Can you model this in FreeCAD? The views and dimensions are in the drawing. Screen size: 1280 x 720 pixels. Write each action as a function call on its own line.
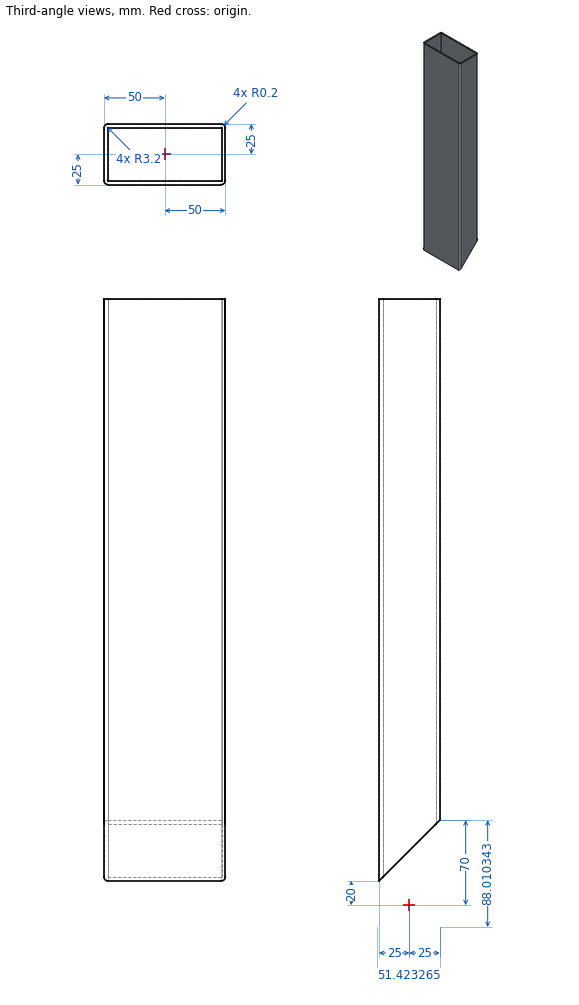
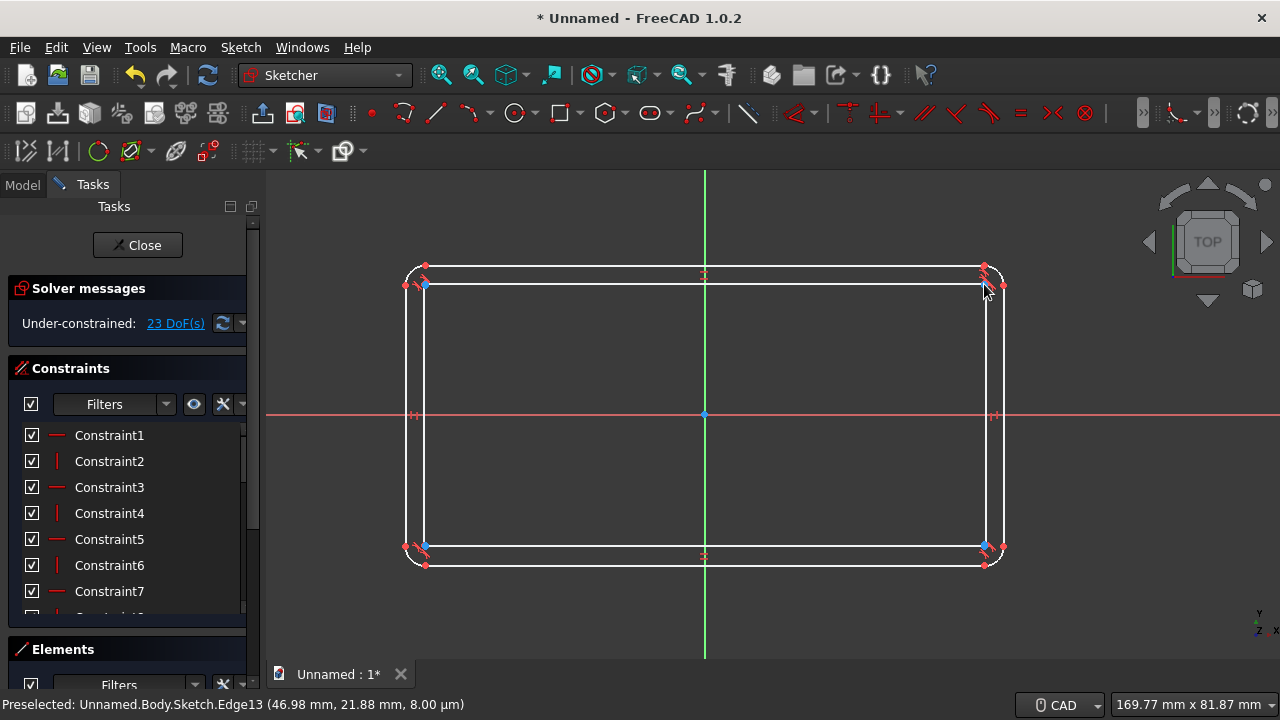
click(593, 284)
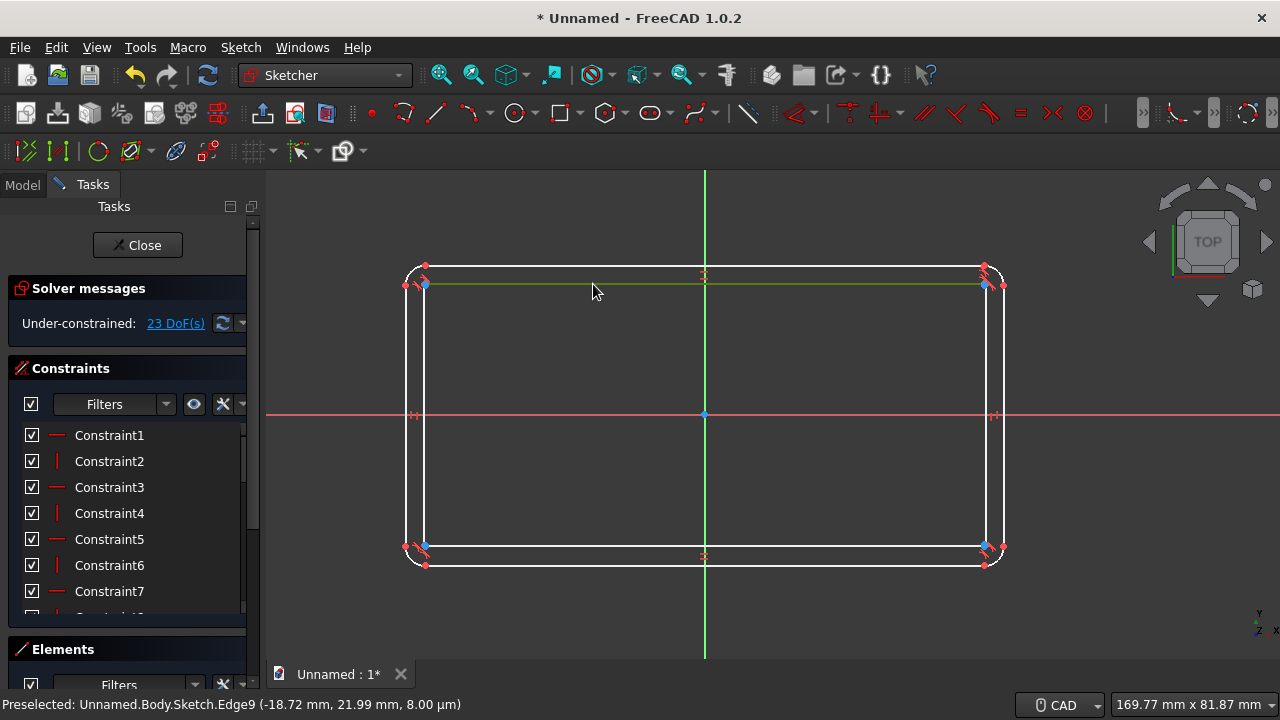
scroll(424, 284, up, 13)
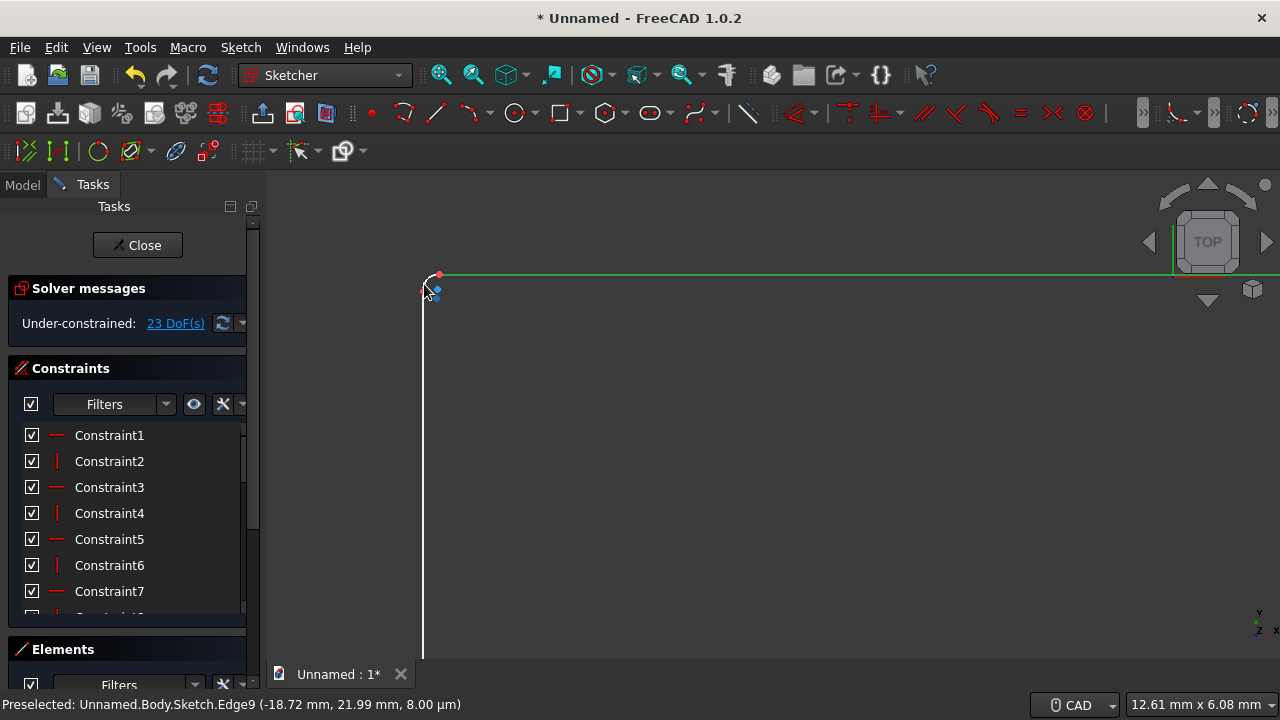
click(427, 279)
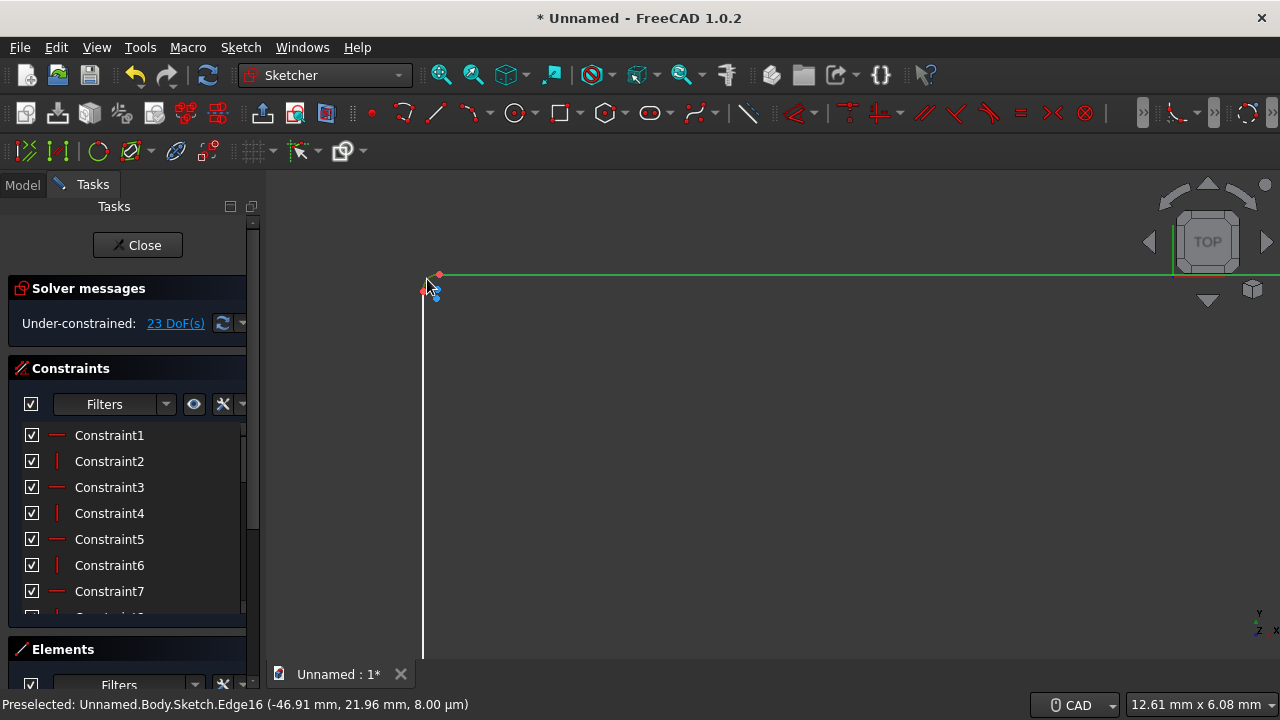
click(990, 114)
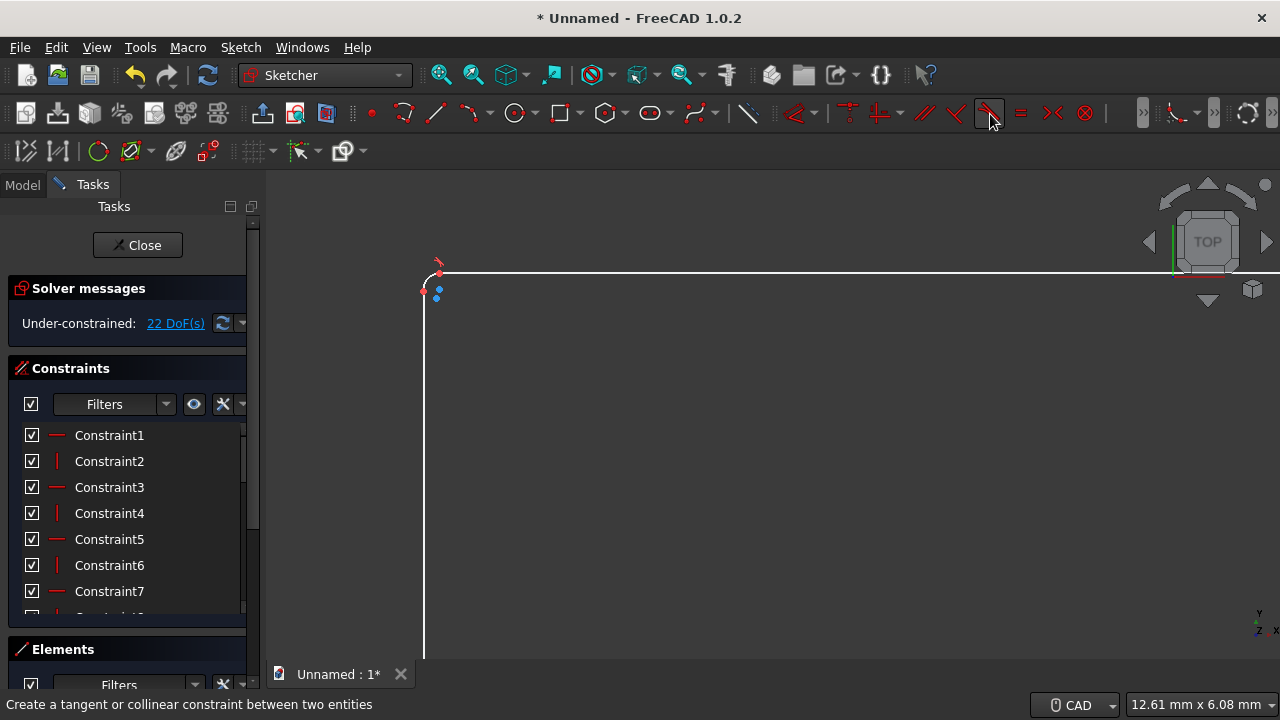
scroll(424, 284, down, 13)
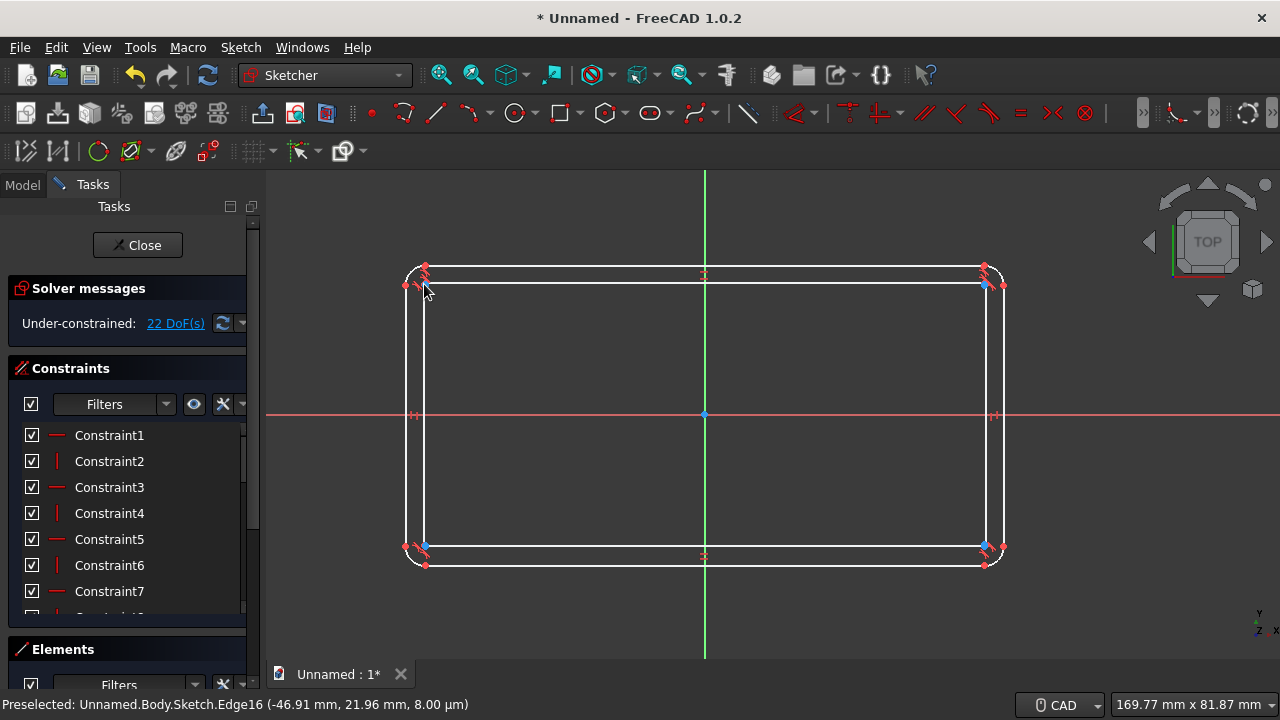
click(986, 363)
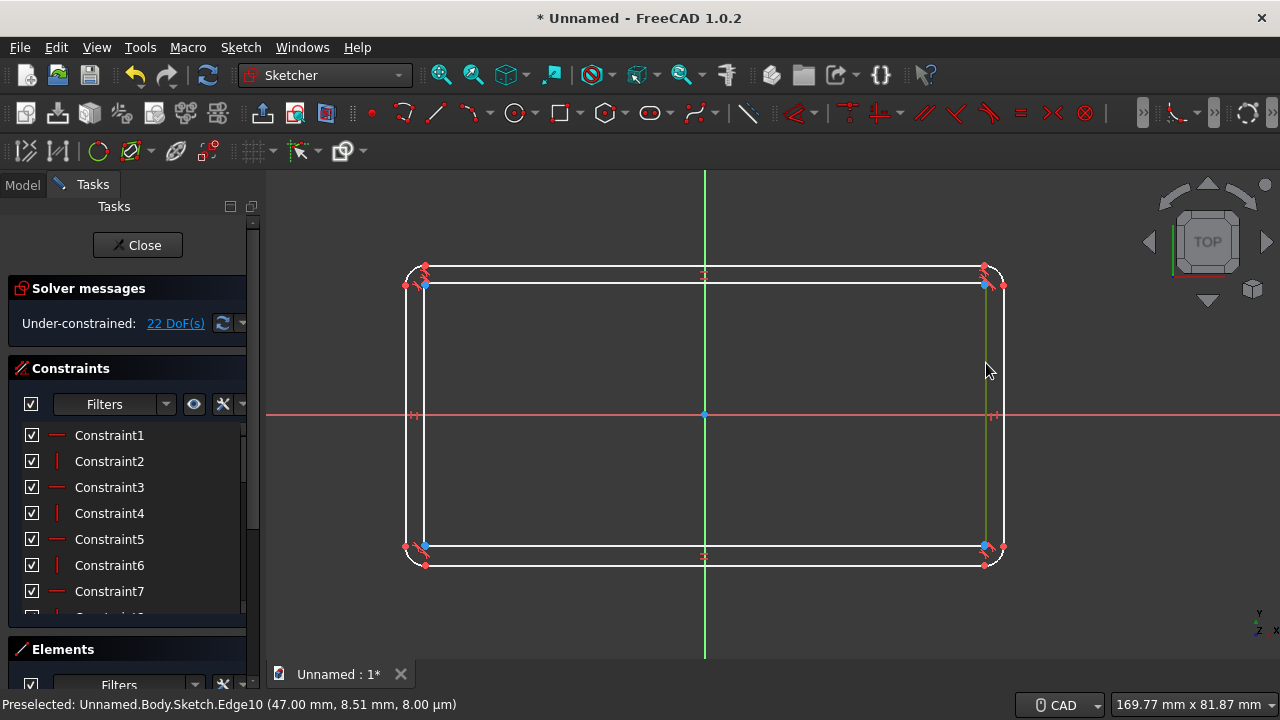
scroll(985, 284, up, 13)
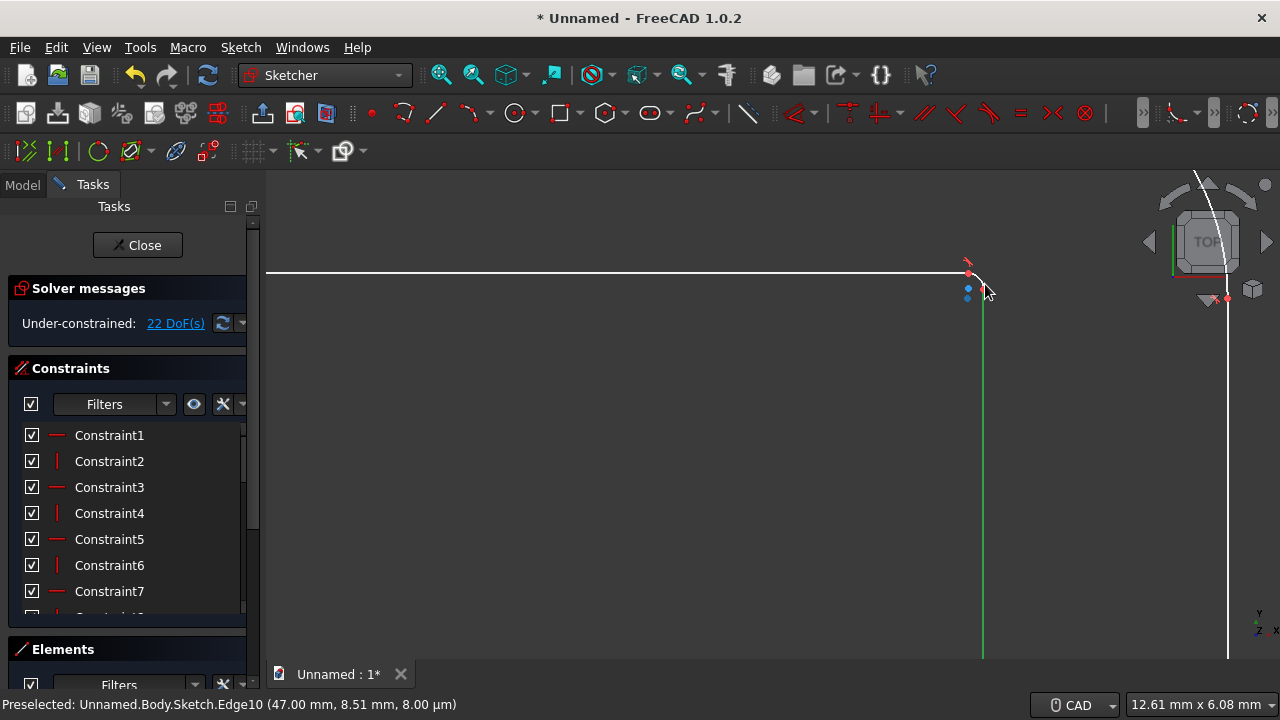
click(979, 278)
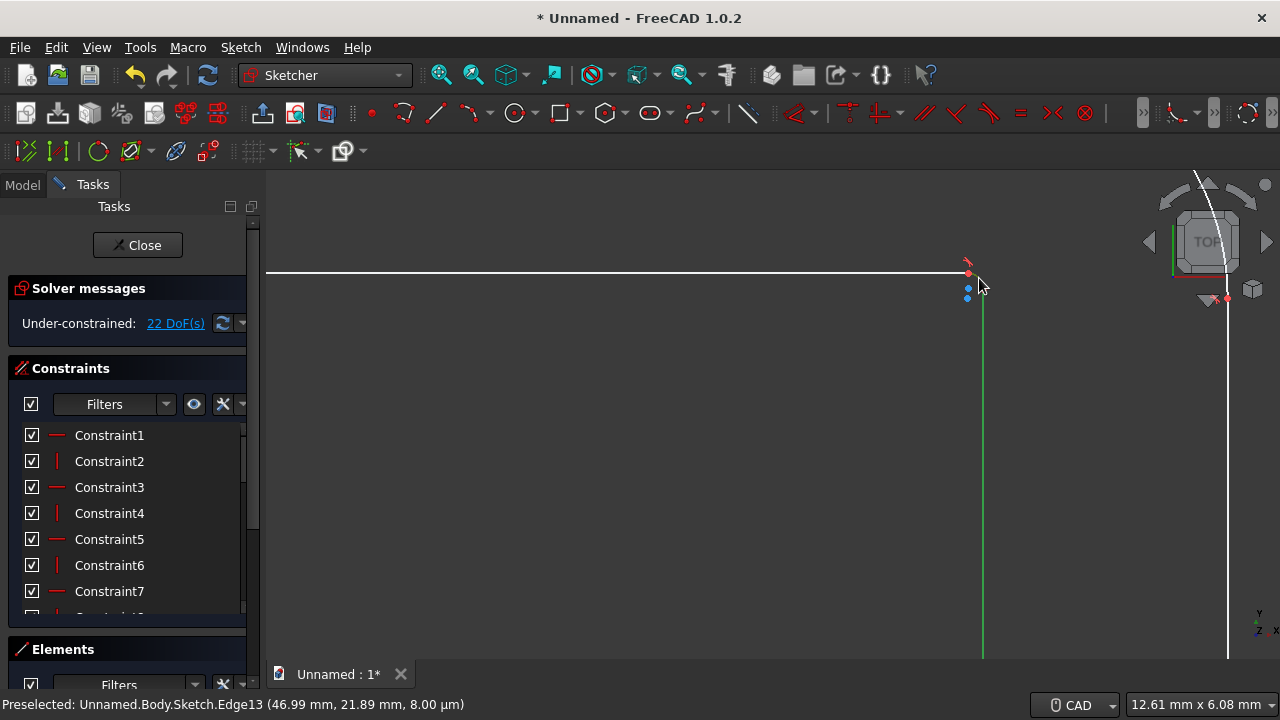
click(990, 114)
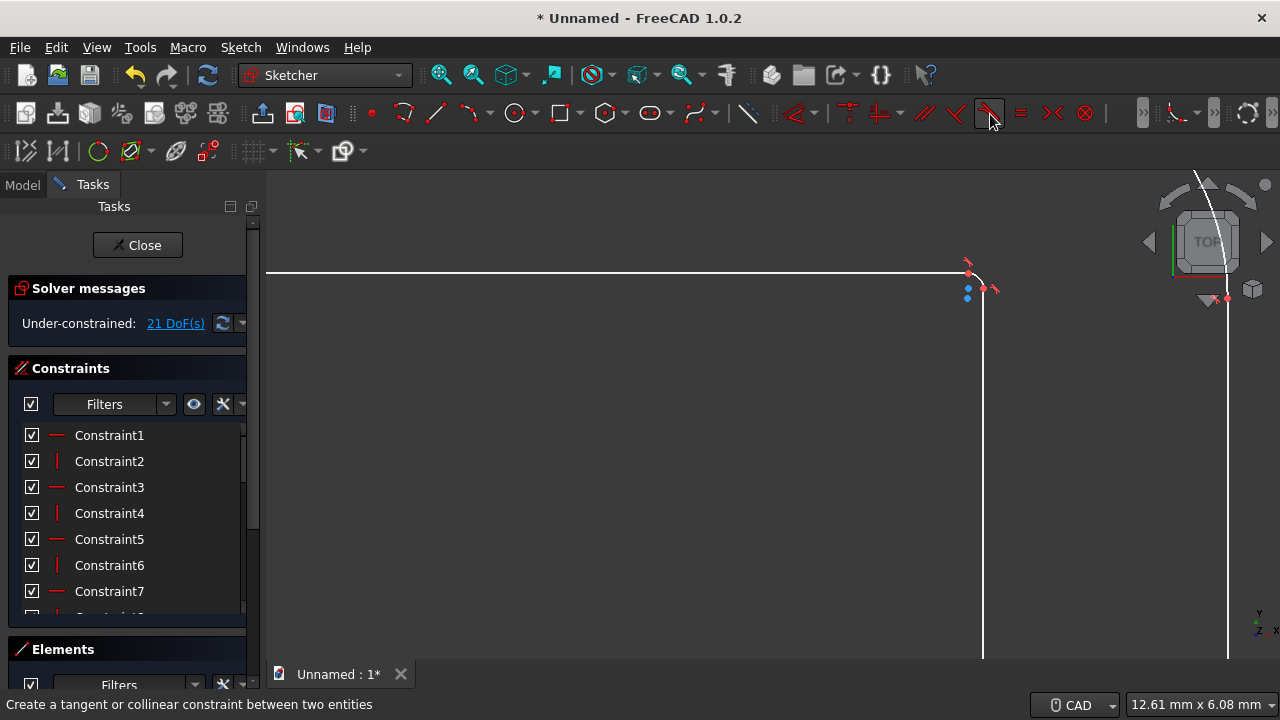
scroll(985, 284, down, 13)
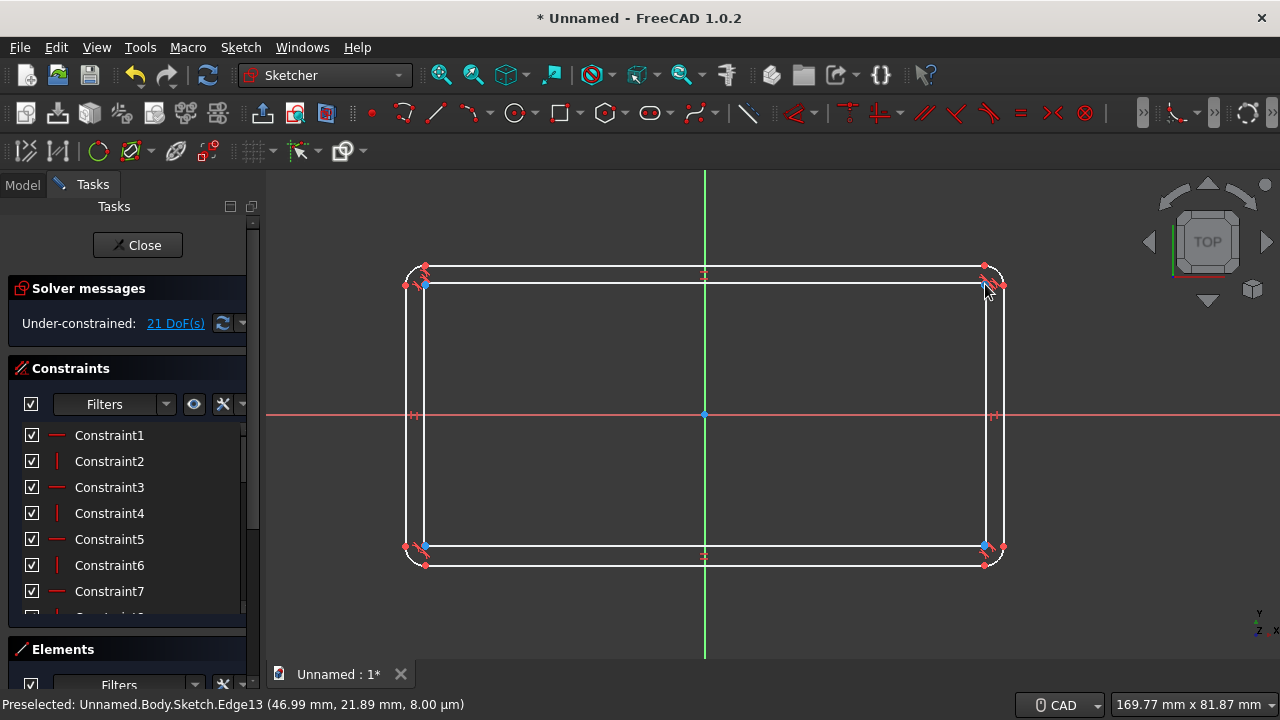
click(986, 363)